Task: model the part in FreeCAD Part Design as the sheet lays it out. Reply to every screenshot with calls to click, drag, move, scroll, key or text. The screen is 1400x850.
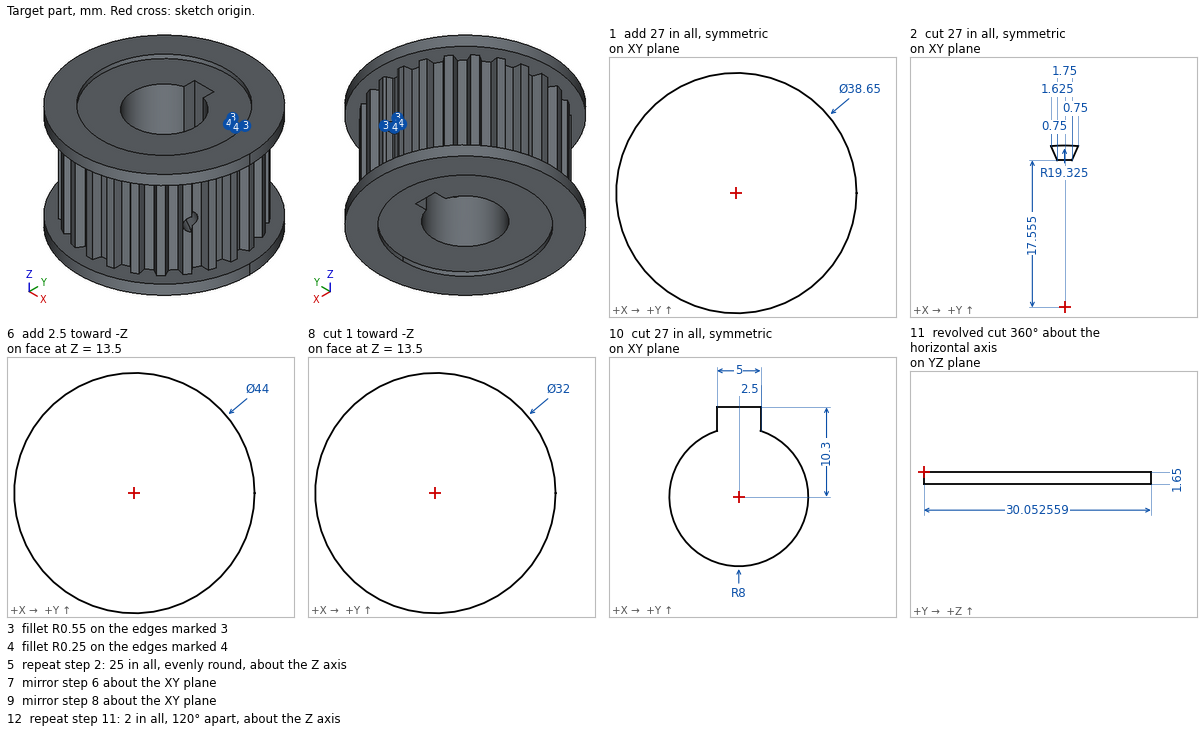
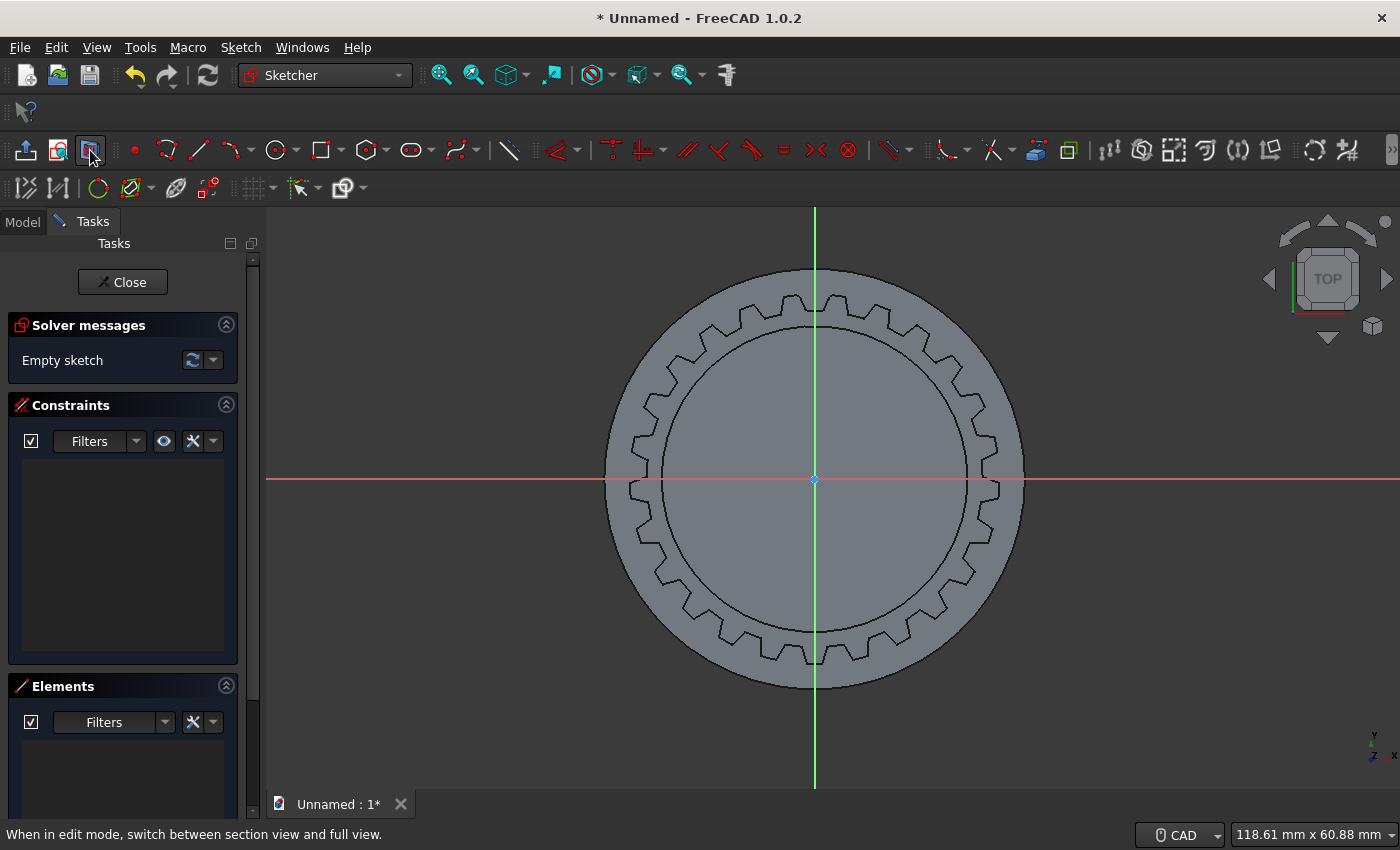
scroll(855, 444, up, 4)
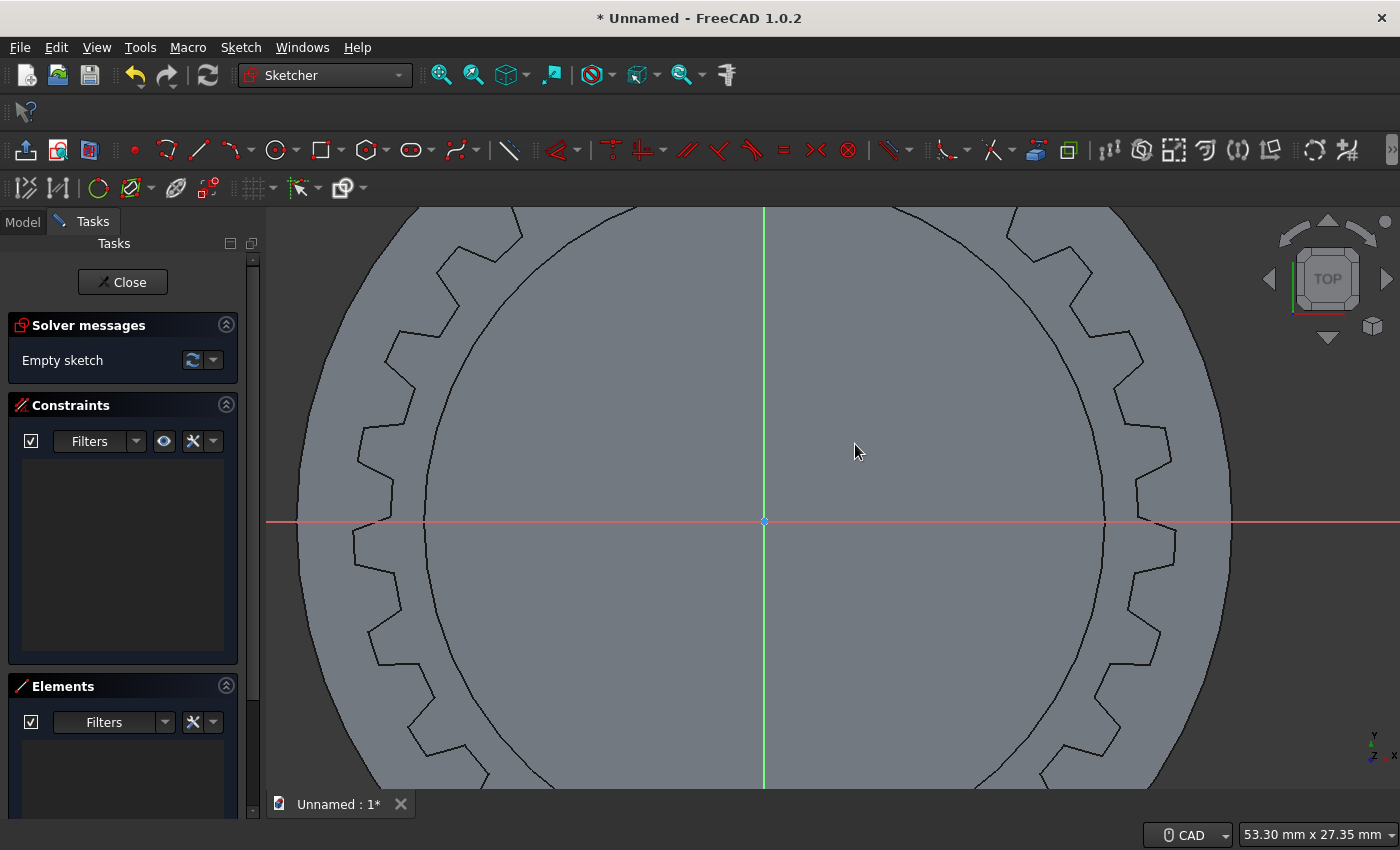
click(168, 150)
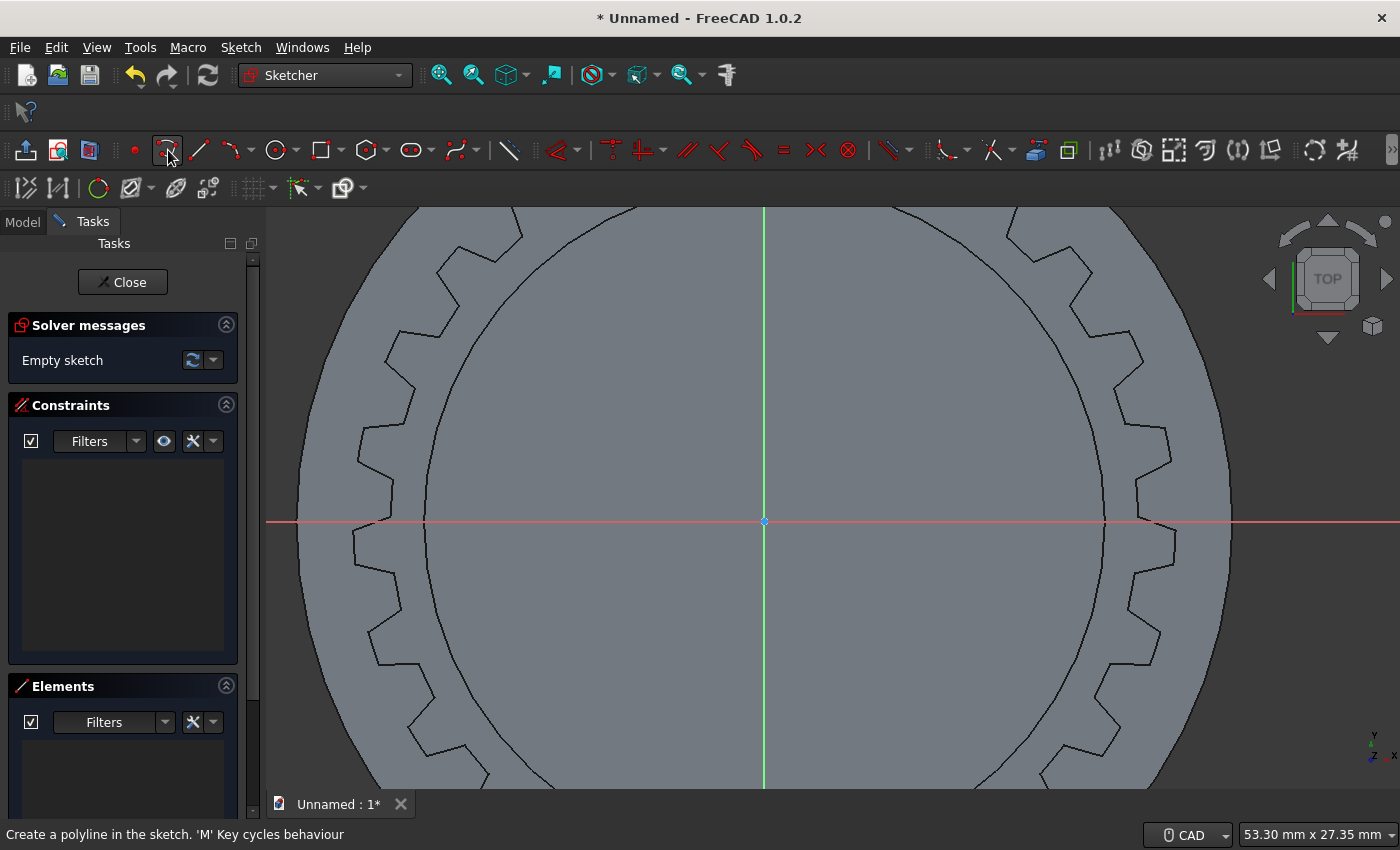
click(818, 360)
click(818, 303)
click(711, 303)
click(711, 360)
right_click(711, 360)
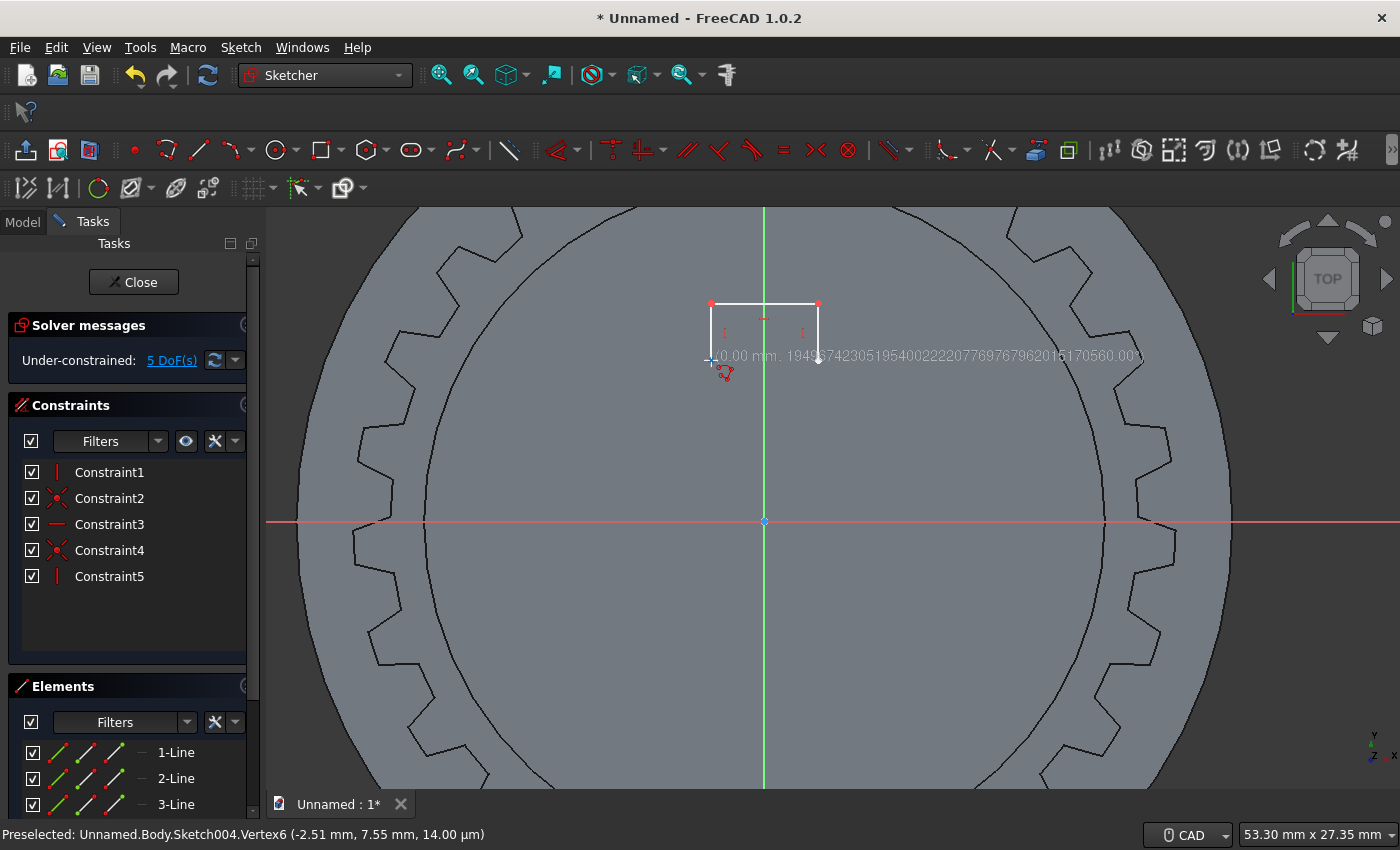
click(232, 150)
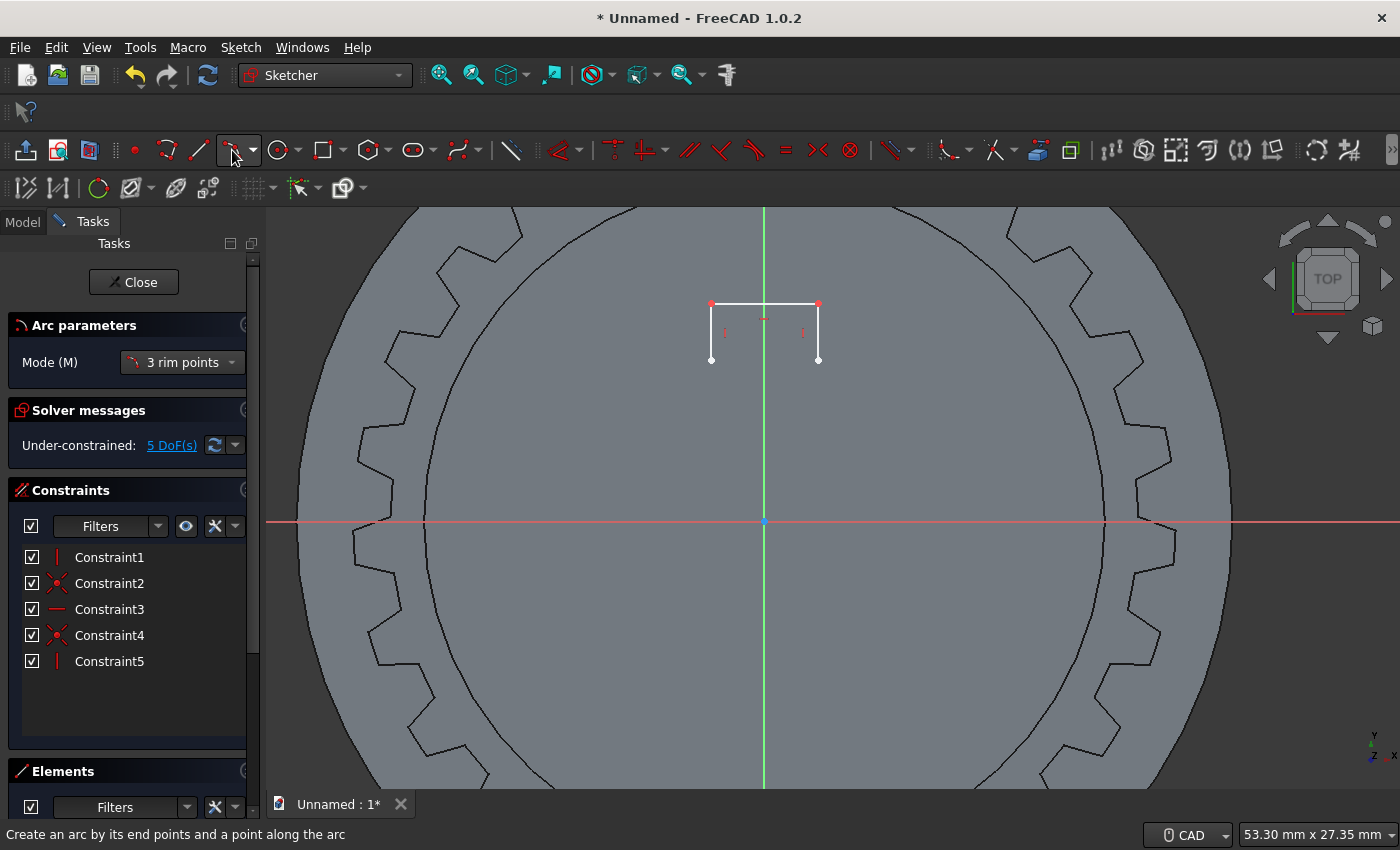
click(711, 361)
click(818, 361)
click(673, 666)
key(Escape)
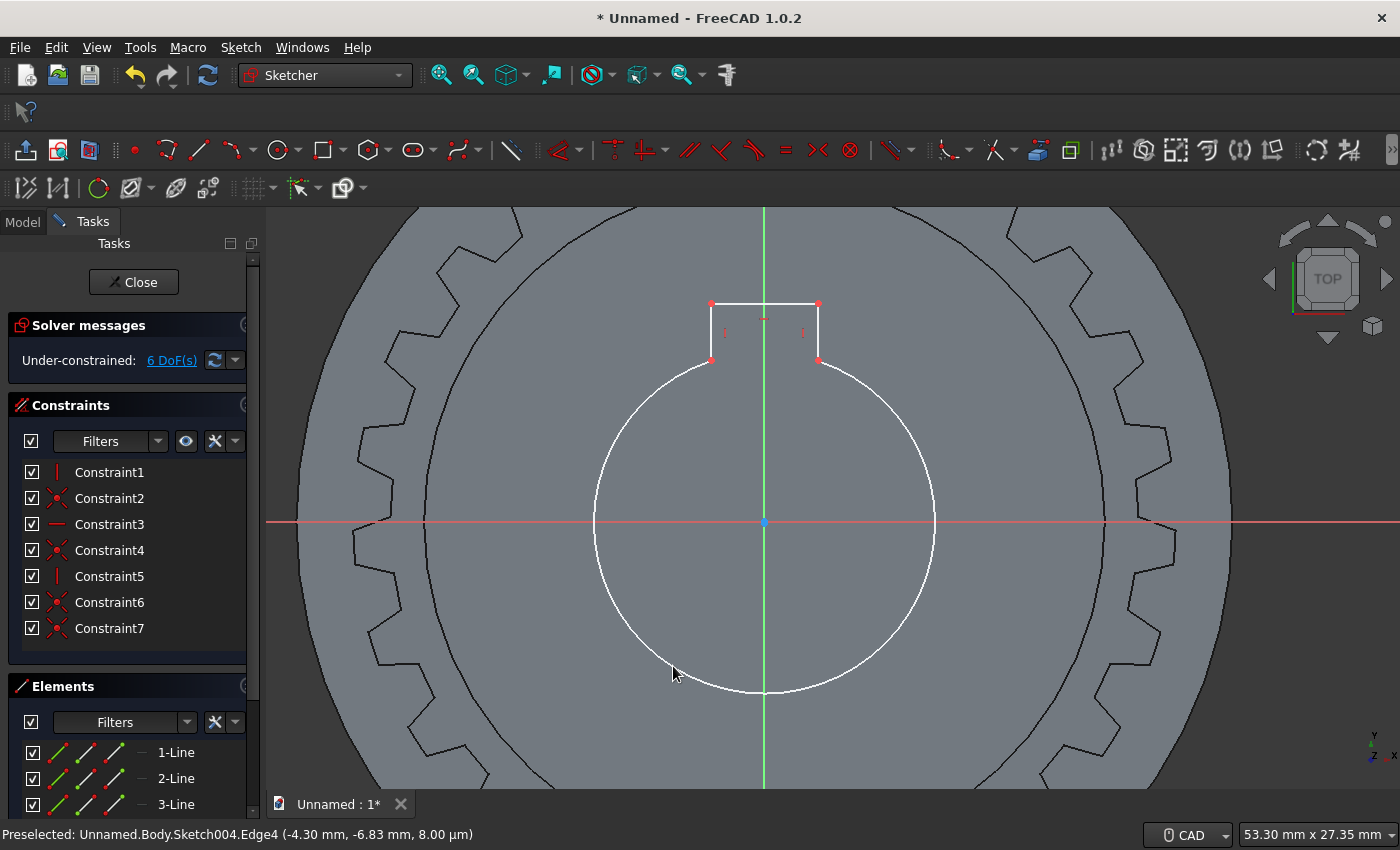
drag(754, 512, 775, 533)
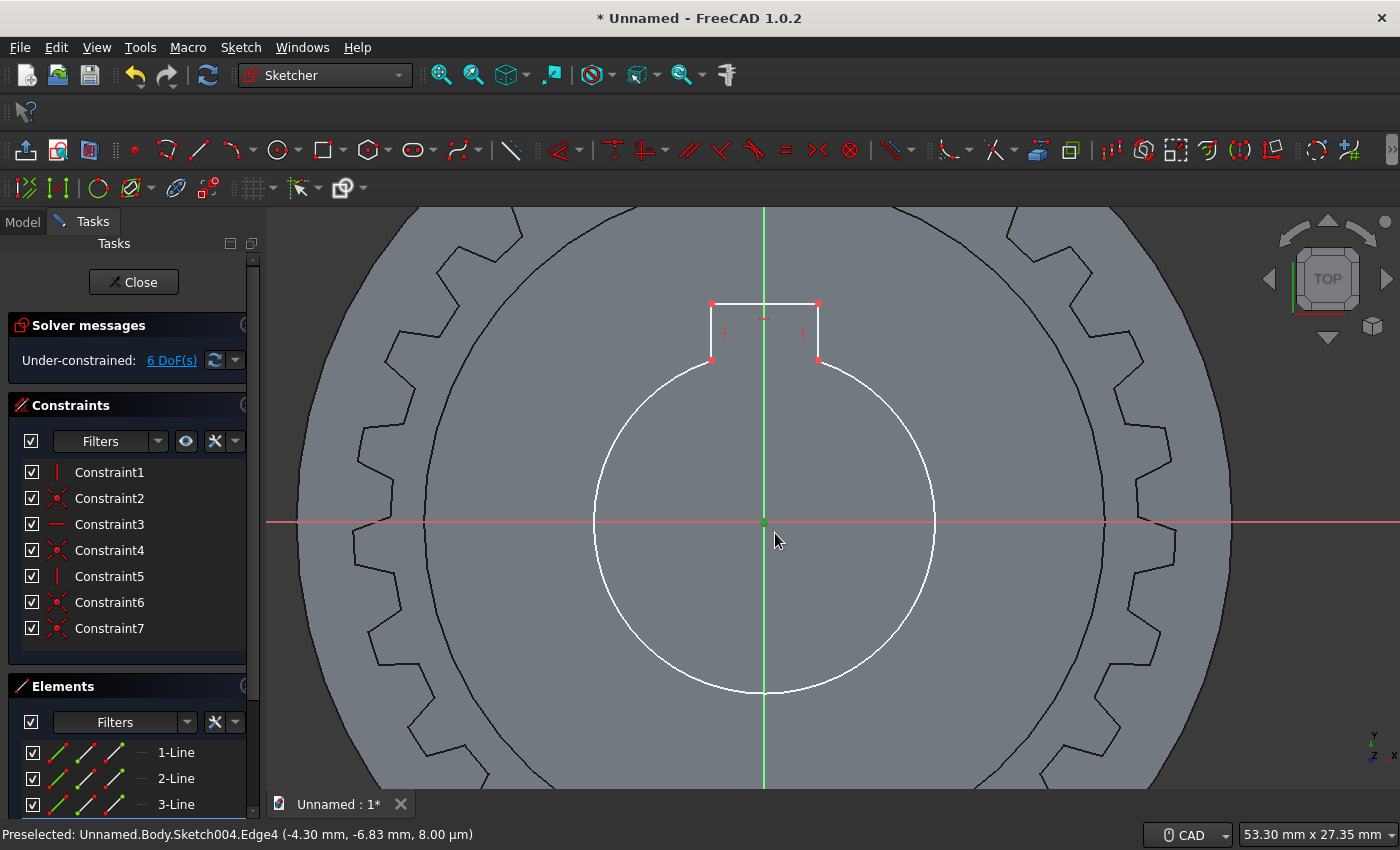
click(614, 150)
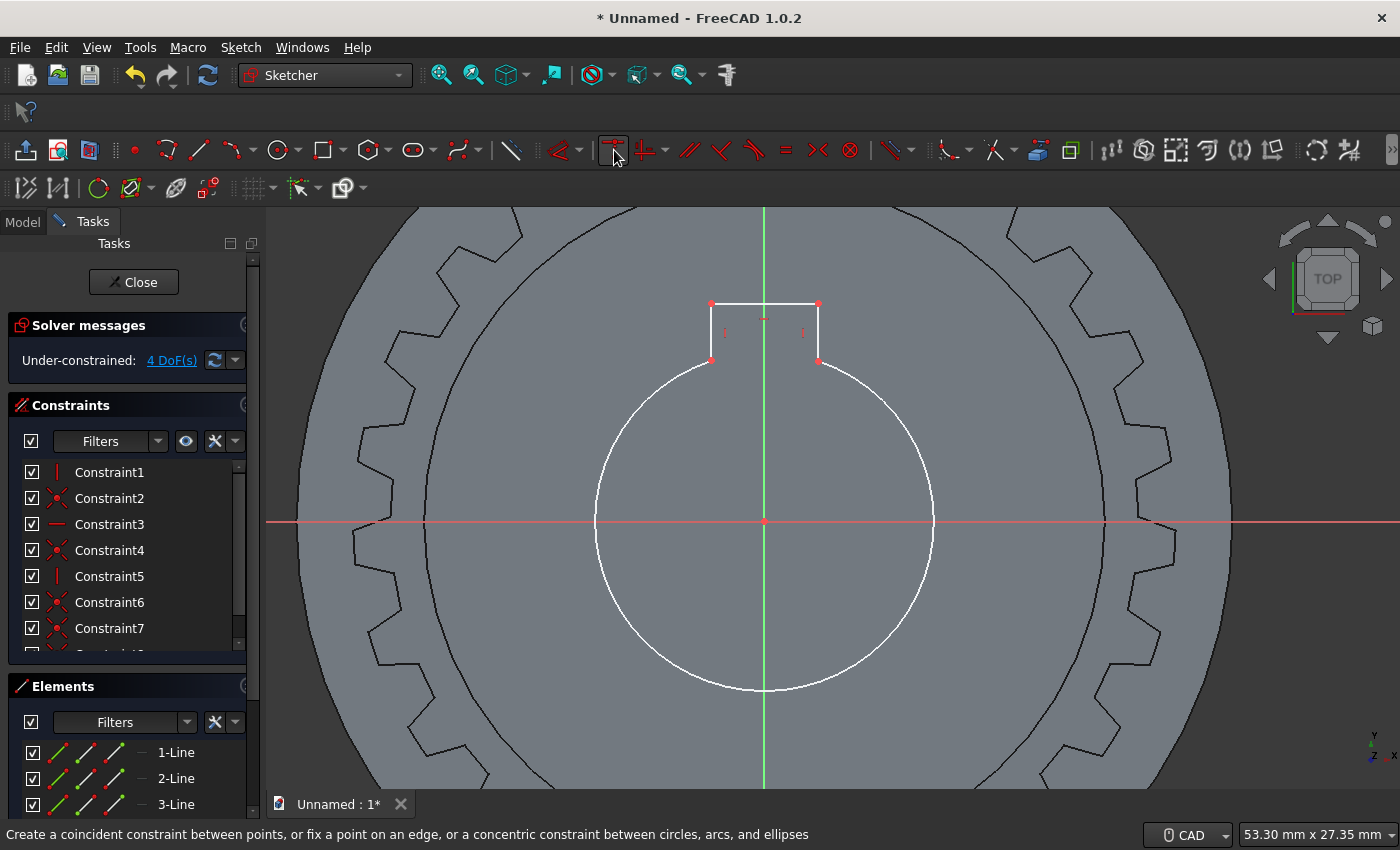
click(558, 150)